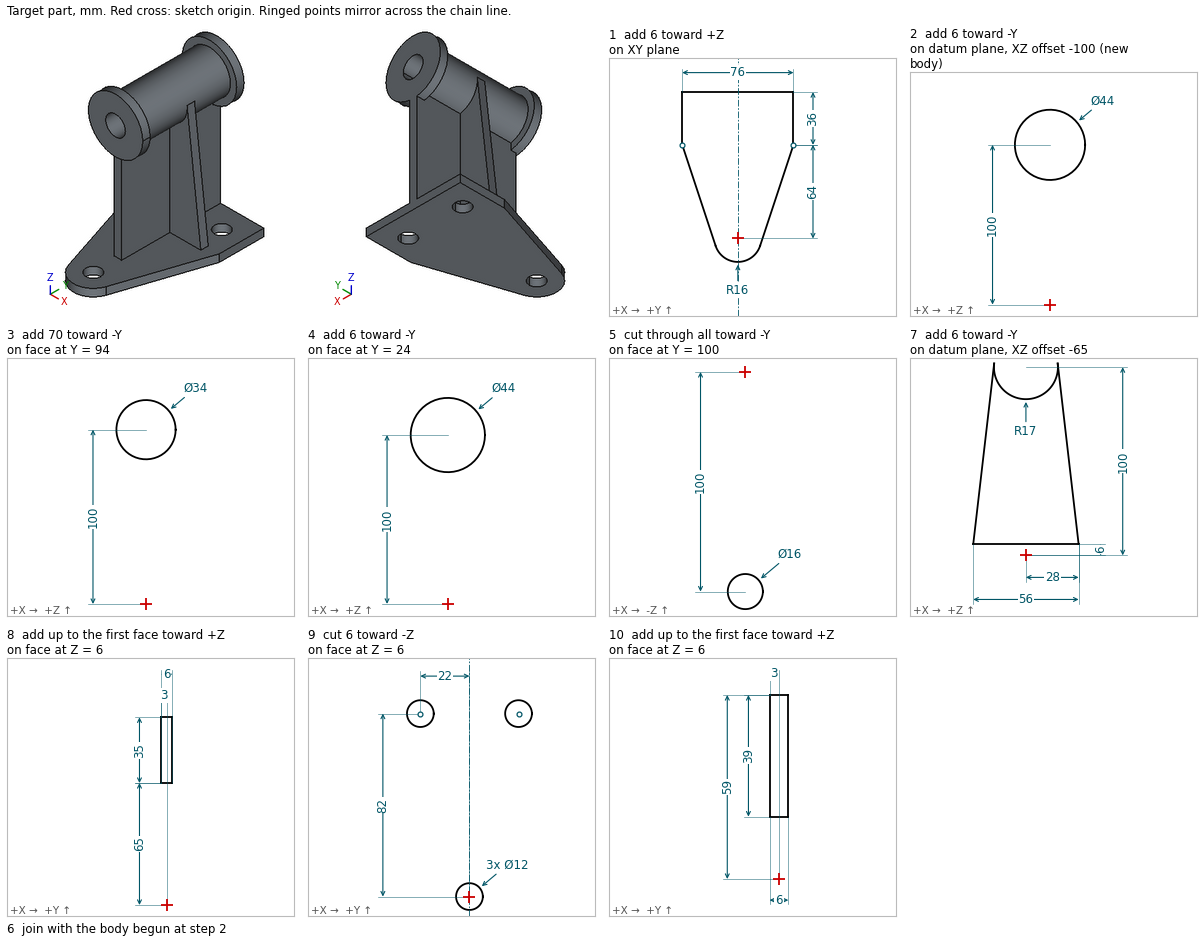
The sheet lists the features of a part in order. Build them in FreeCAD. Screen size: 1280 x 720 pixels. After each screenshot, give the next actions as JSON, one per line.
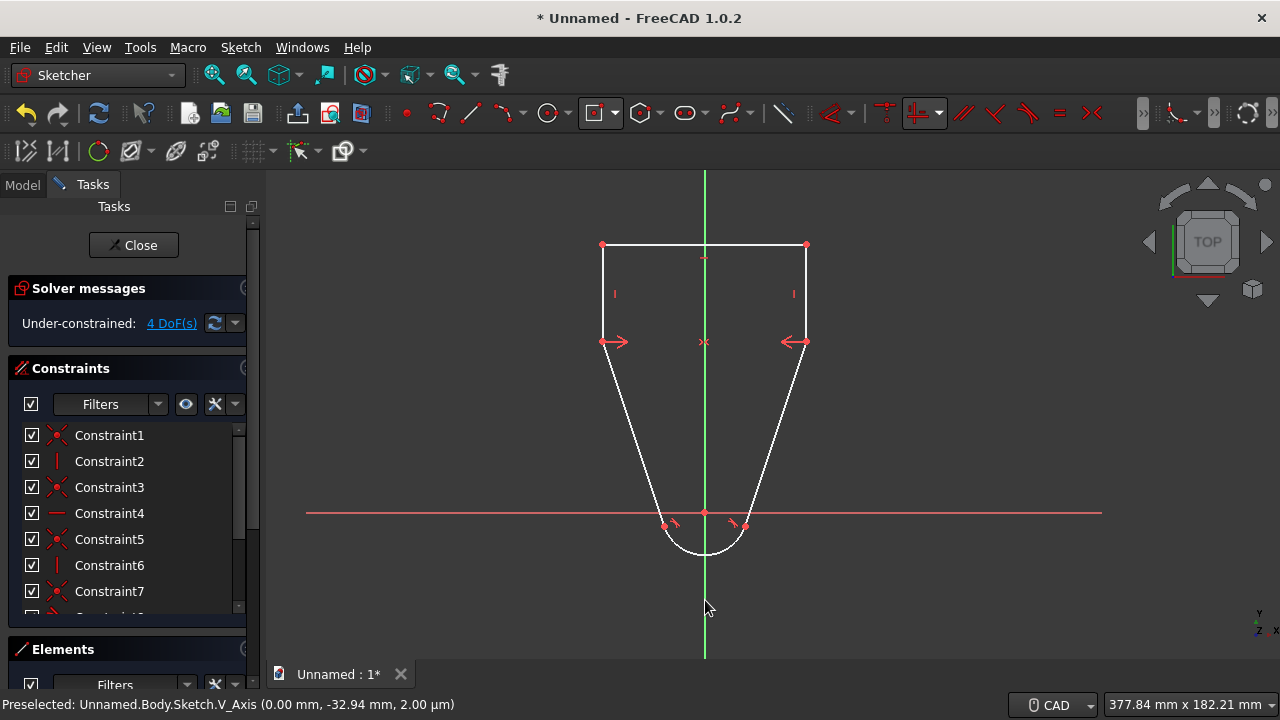
{"action": "left_click", "coordinate": [684, 550]}
{"action": "left_click", "coordinate": [669, 578]}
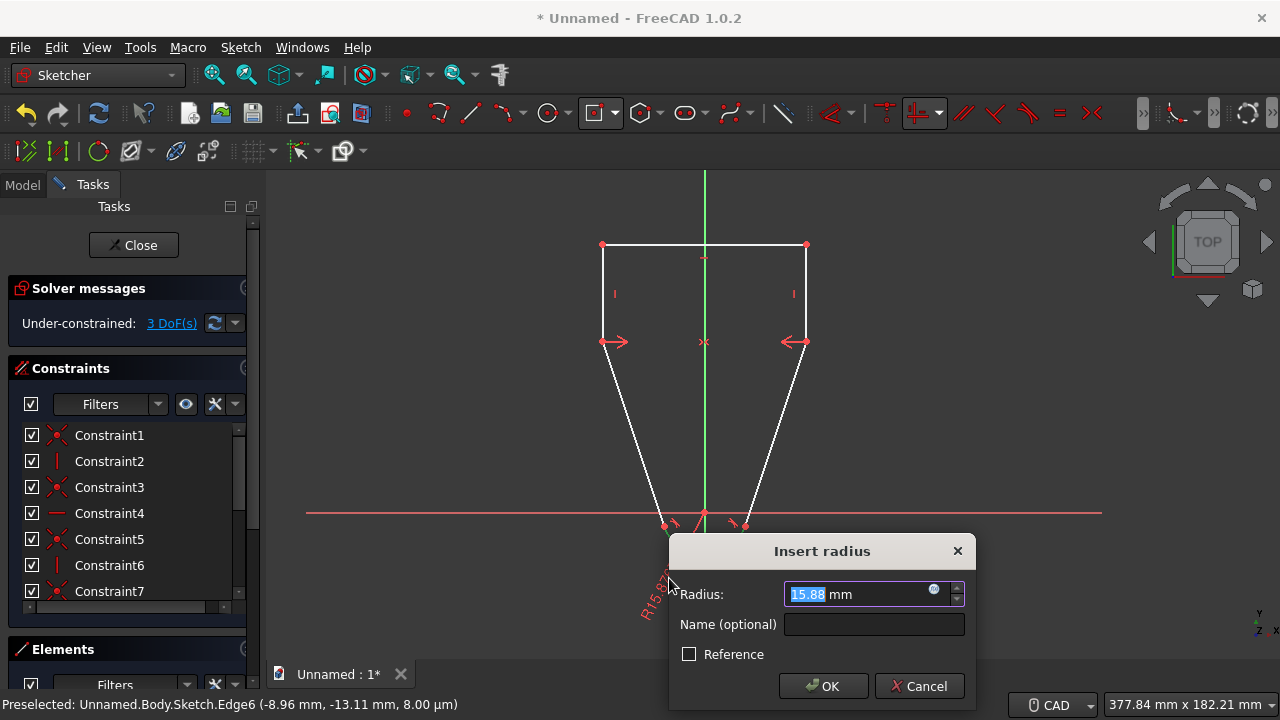
{"action": "type", "text": "16"}
{"action": "key", "text": "Return"}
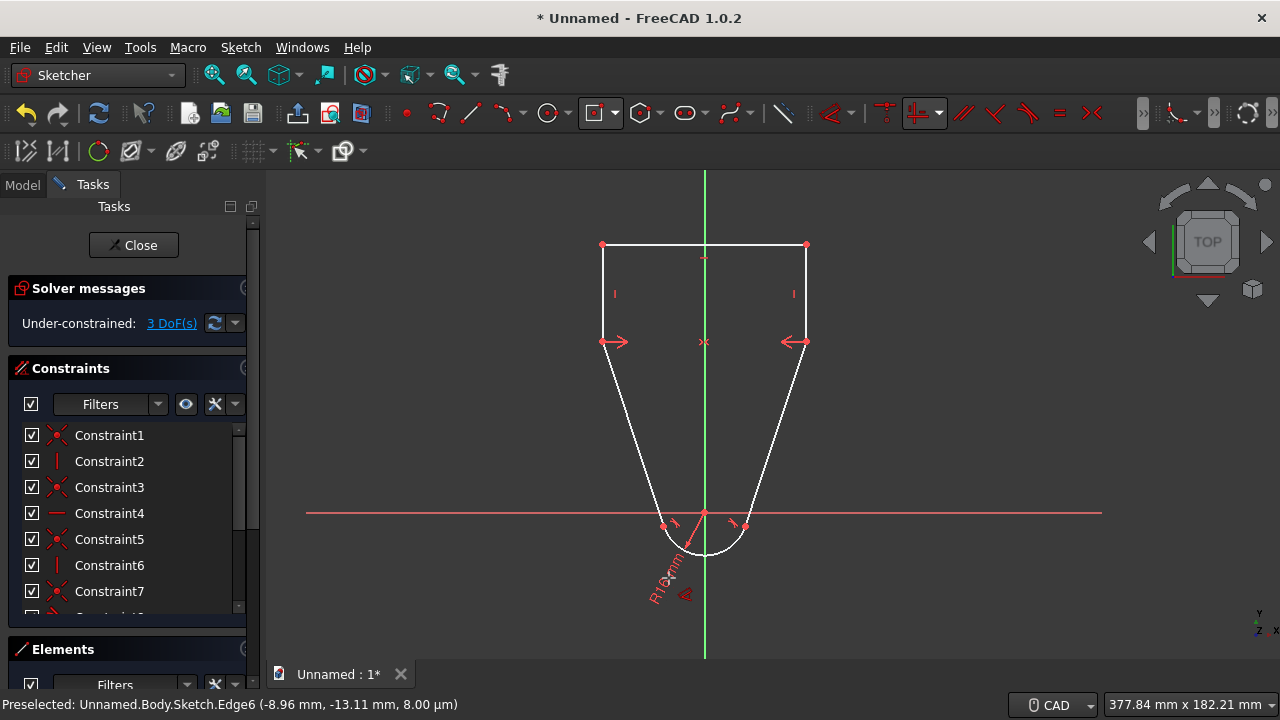
{"action": "left_click", "coordinate": [806, 313]}
{"action": "left_click", "coordinate": [840, 293]}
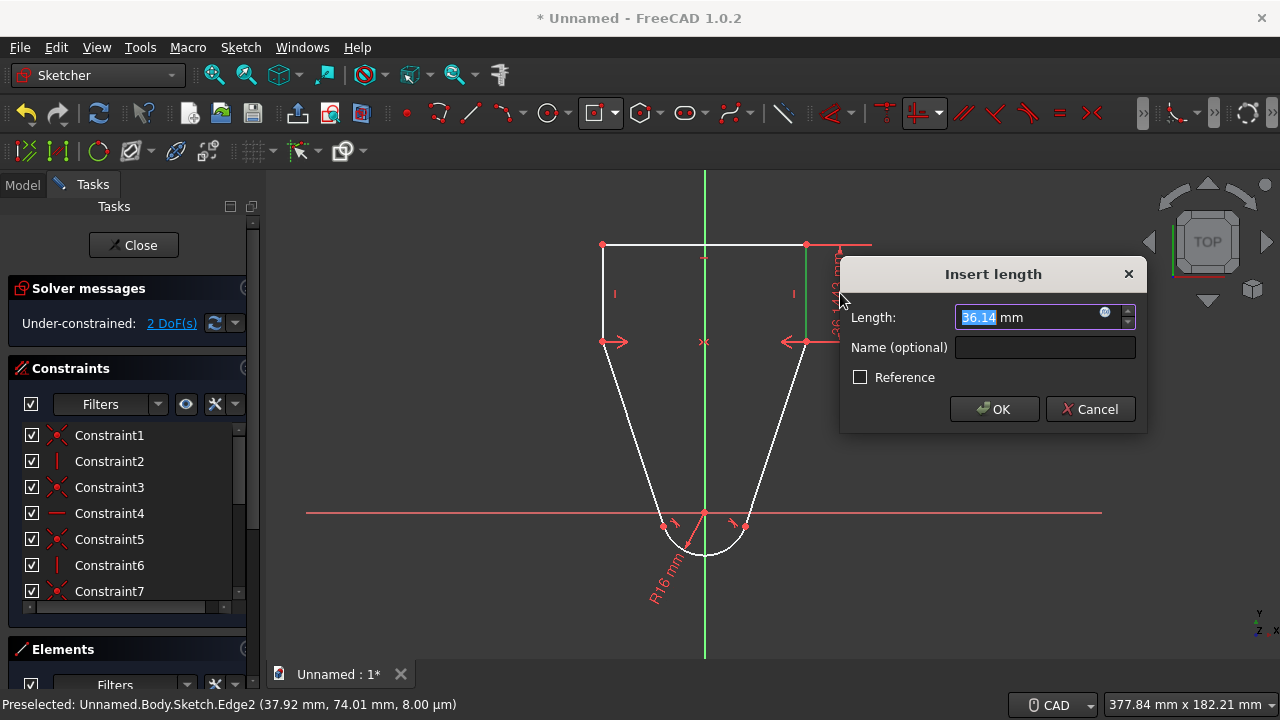
{"action": "type", "text": "36"}
{"action": "key", "text": "Return"}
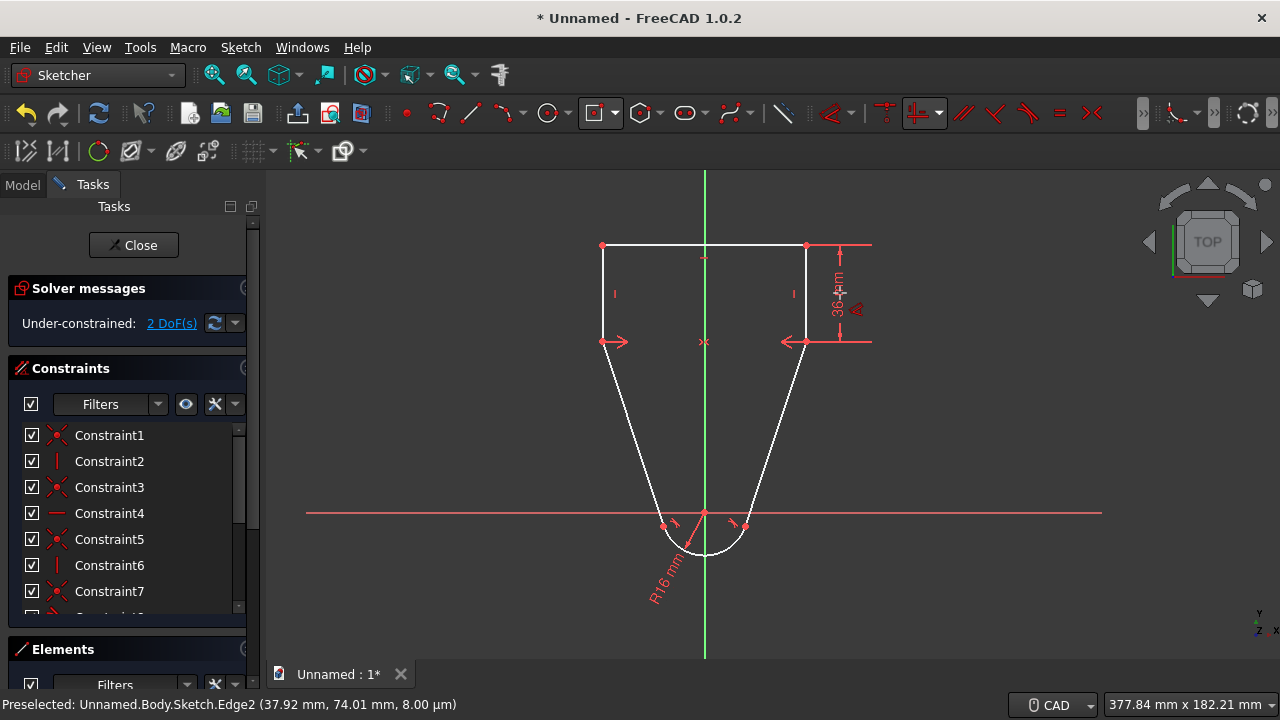
{"action": "left_click", "coordinate": [745, 245]}
{"action": "left_click", "coordinate": [658, 211]}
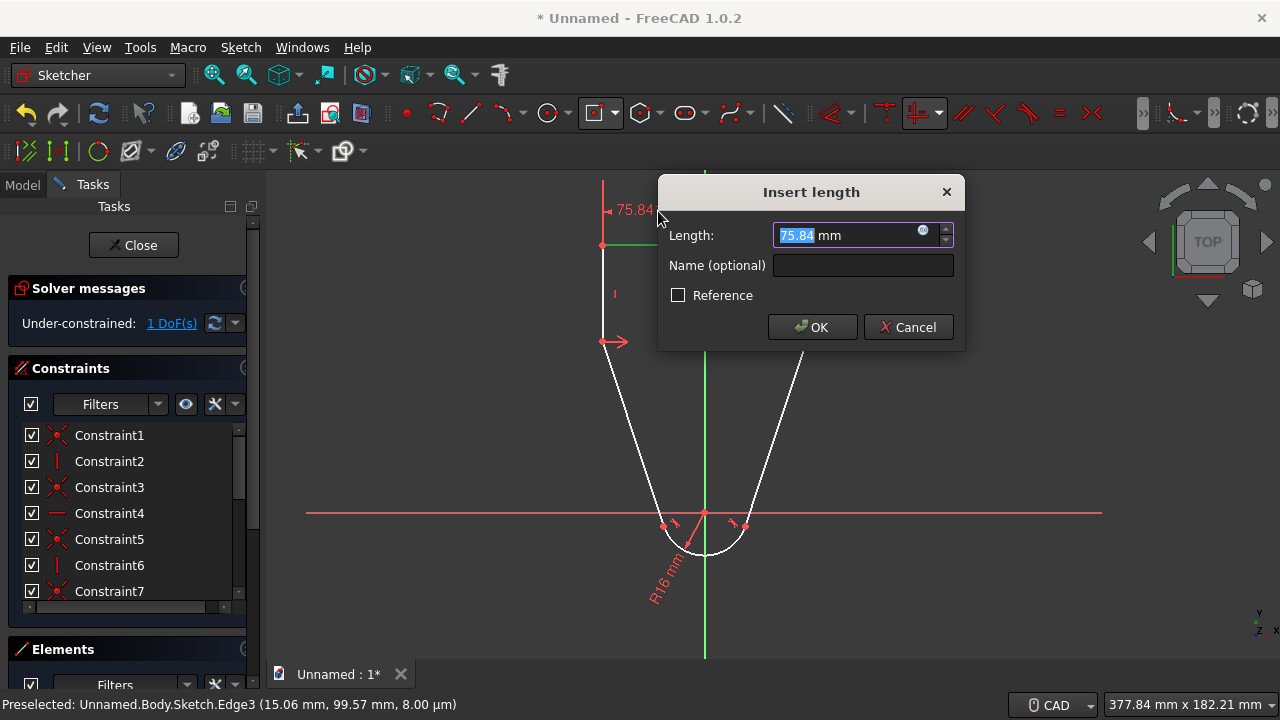
{"action": "type", "text": "76"}
{"action": "key", "text": "Return"}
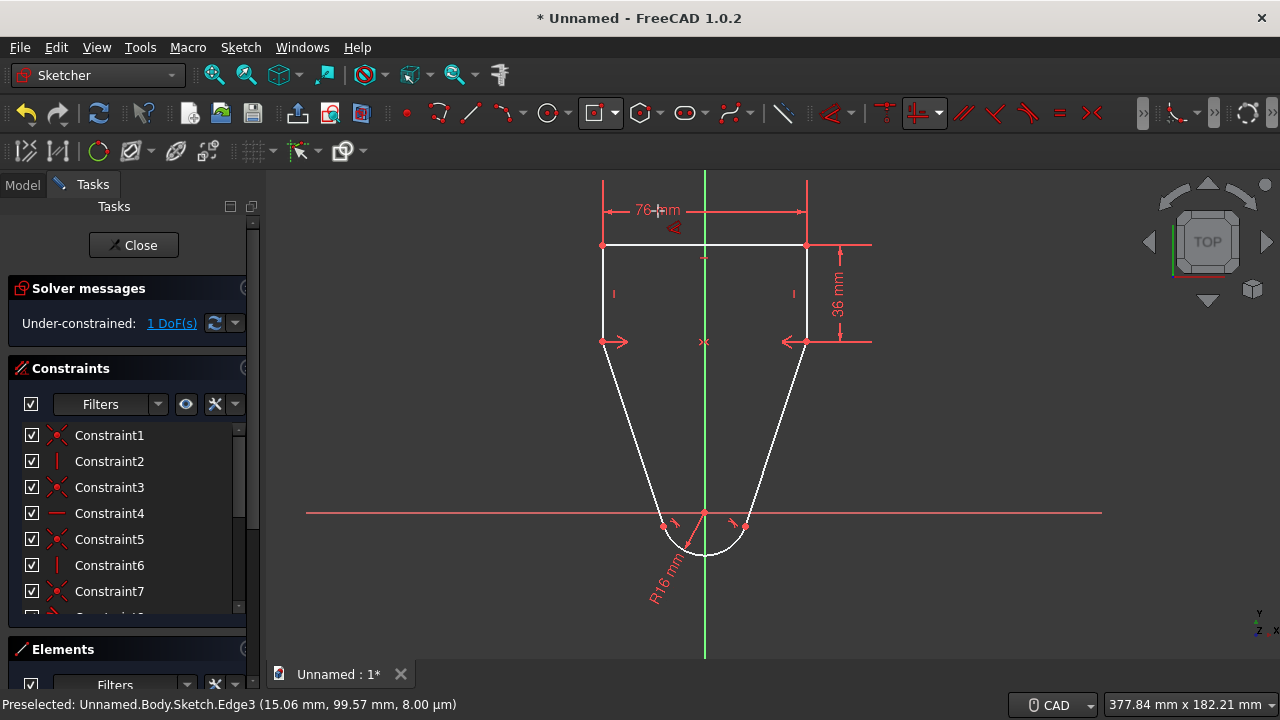
{"action": "left_click", "coordinate": [807, 342]}
{"action": "left_click", "coordinate": [841, 427]}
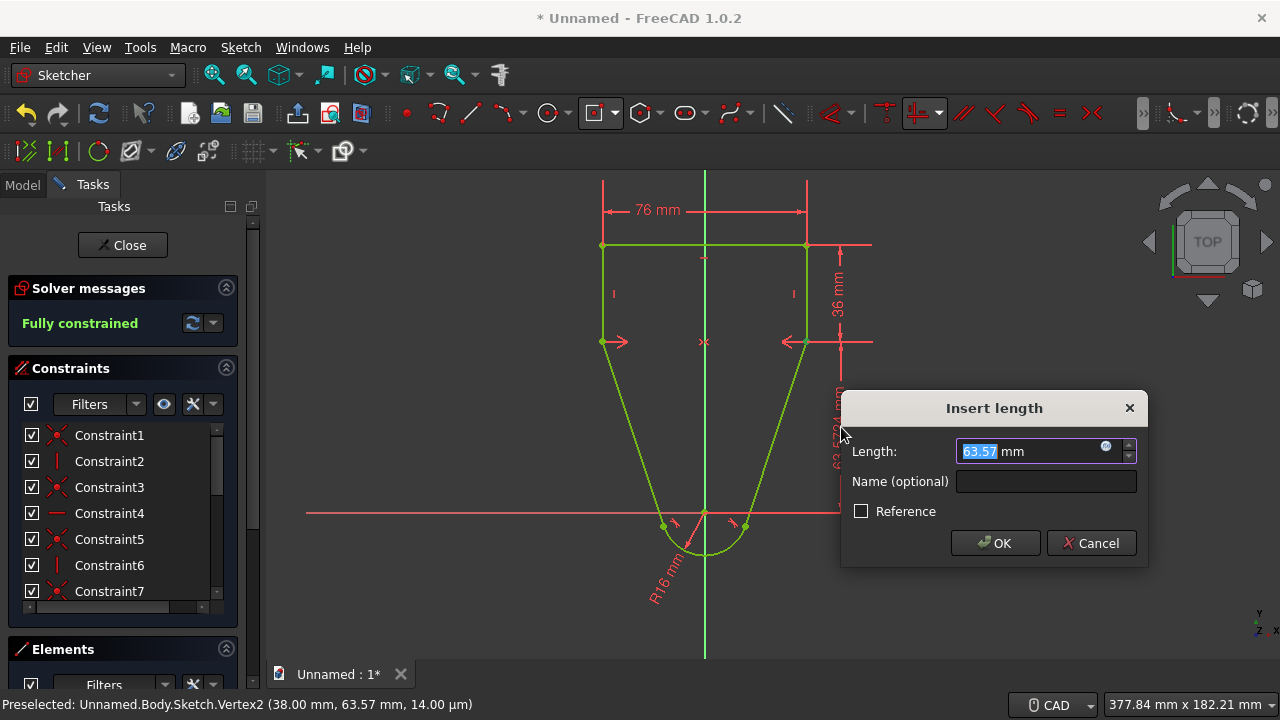
{"action": "type", "text": "64"}
{"action": "key", "text": "Return"}
{"action": "key", "text": "Escape"}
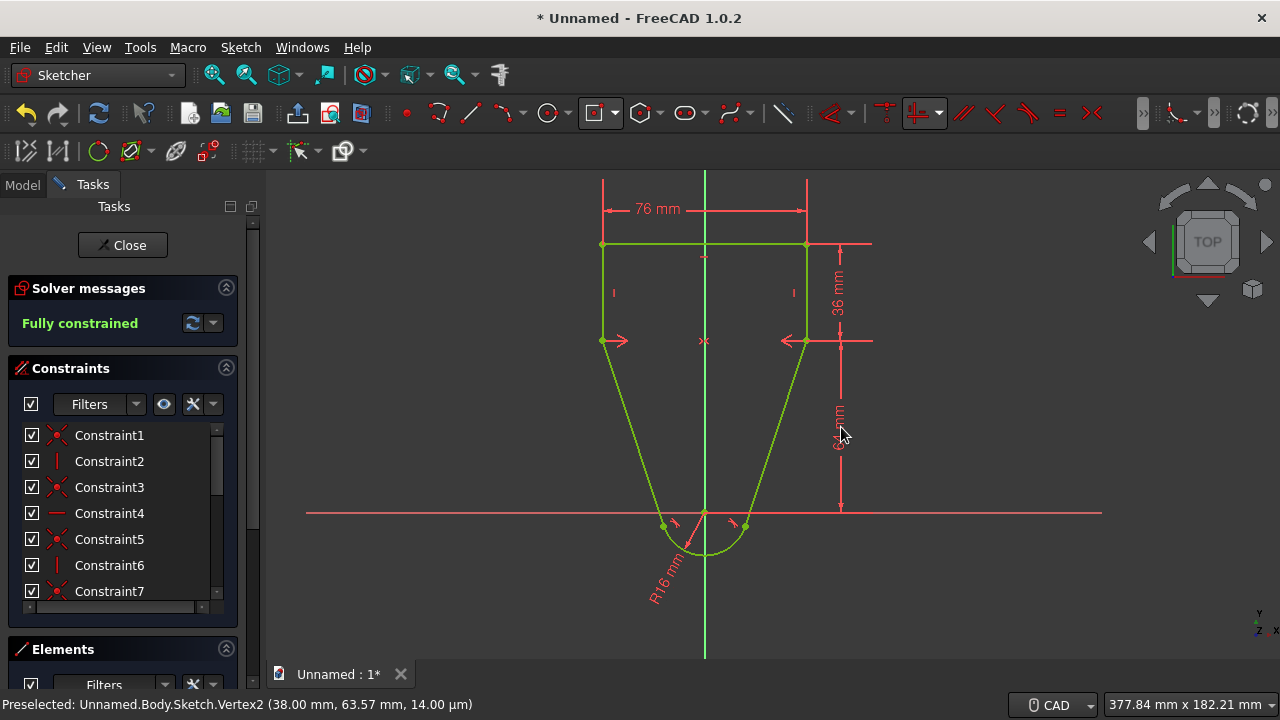
{"action": "left_click", "coordinate": [123, 245]}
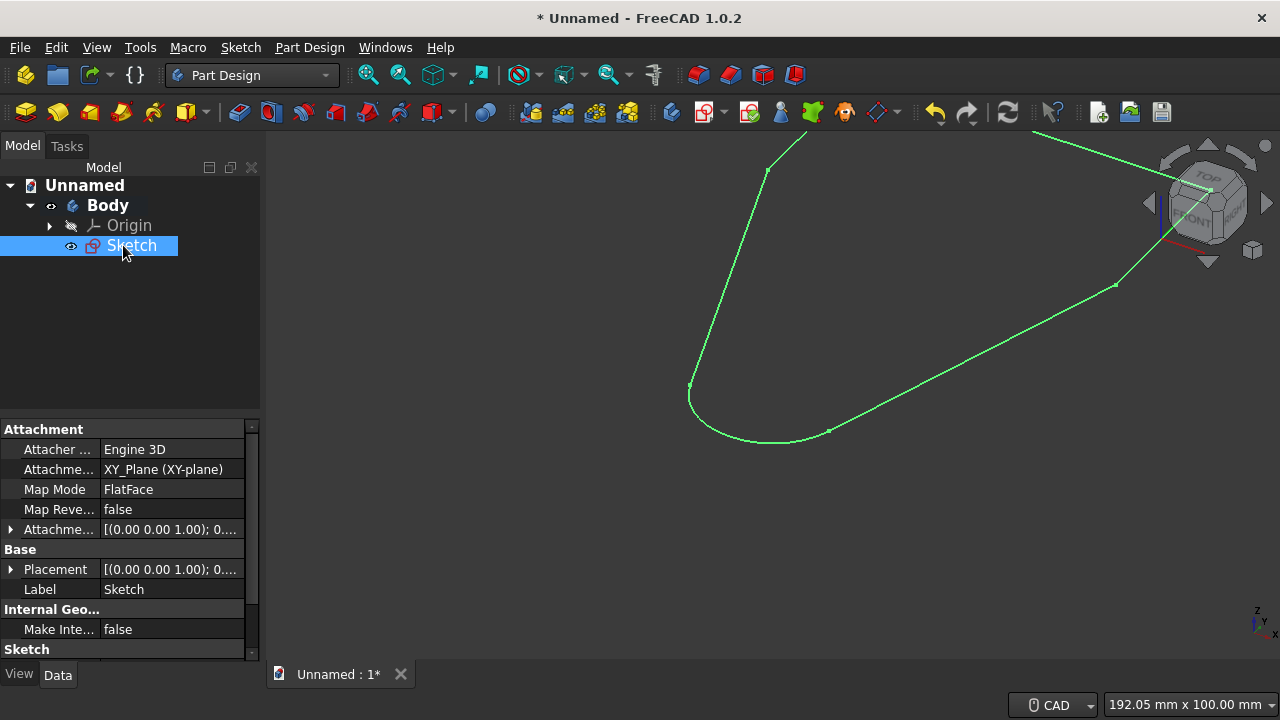
{"action": "left_click", "coordinate": [26, 112]}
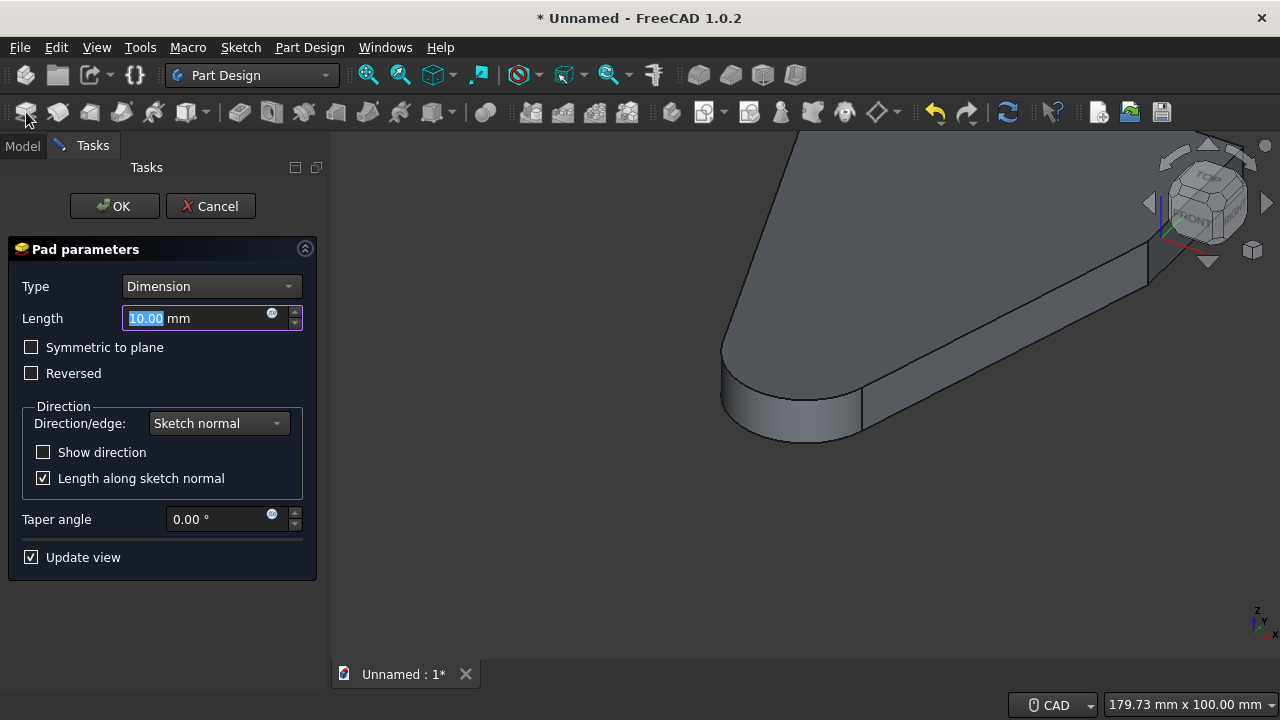
{"action": "type", "text": "6"}
{"action": "key", "text": "Tab"}